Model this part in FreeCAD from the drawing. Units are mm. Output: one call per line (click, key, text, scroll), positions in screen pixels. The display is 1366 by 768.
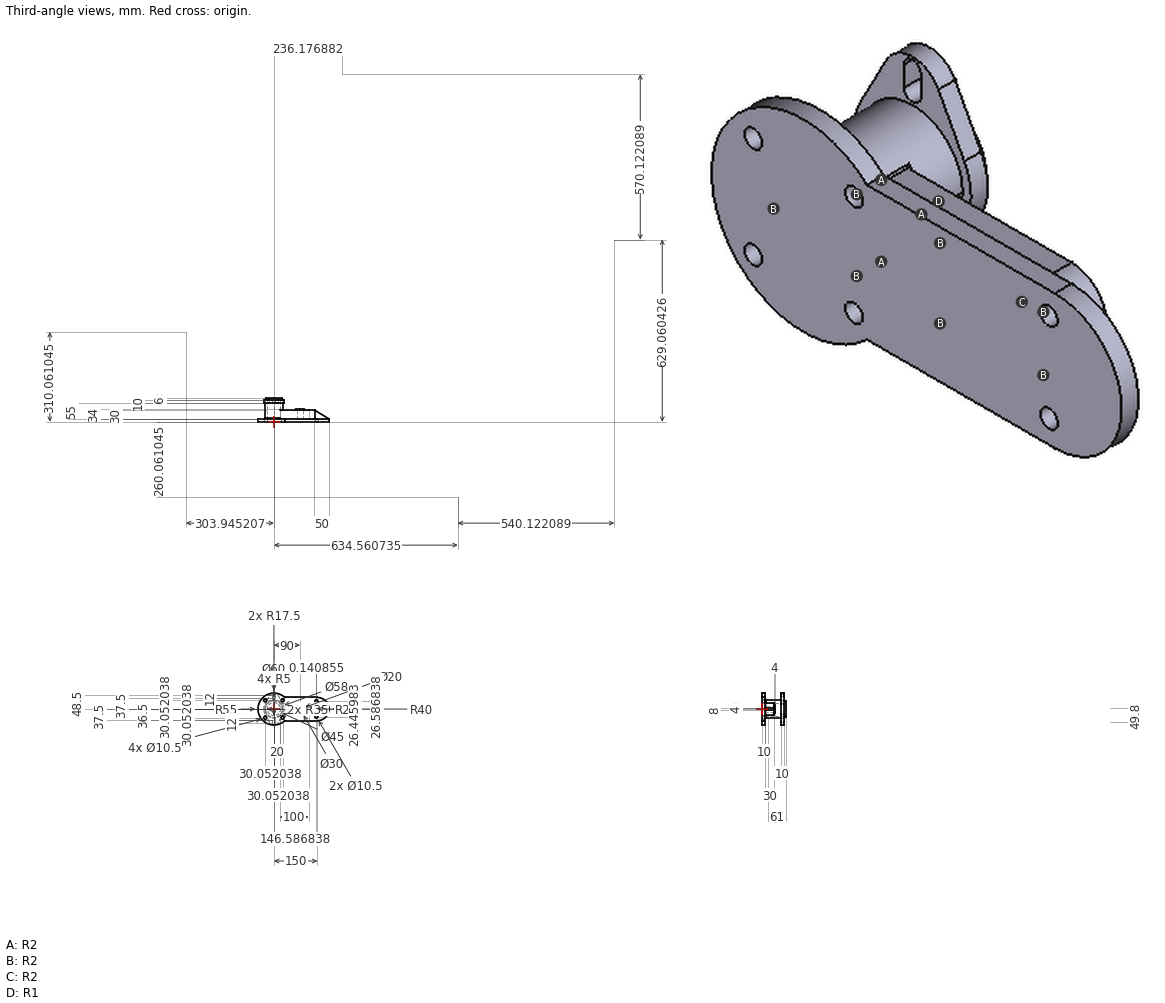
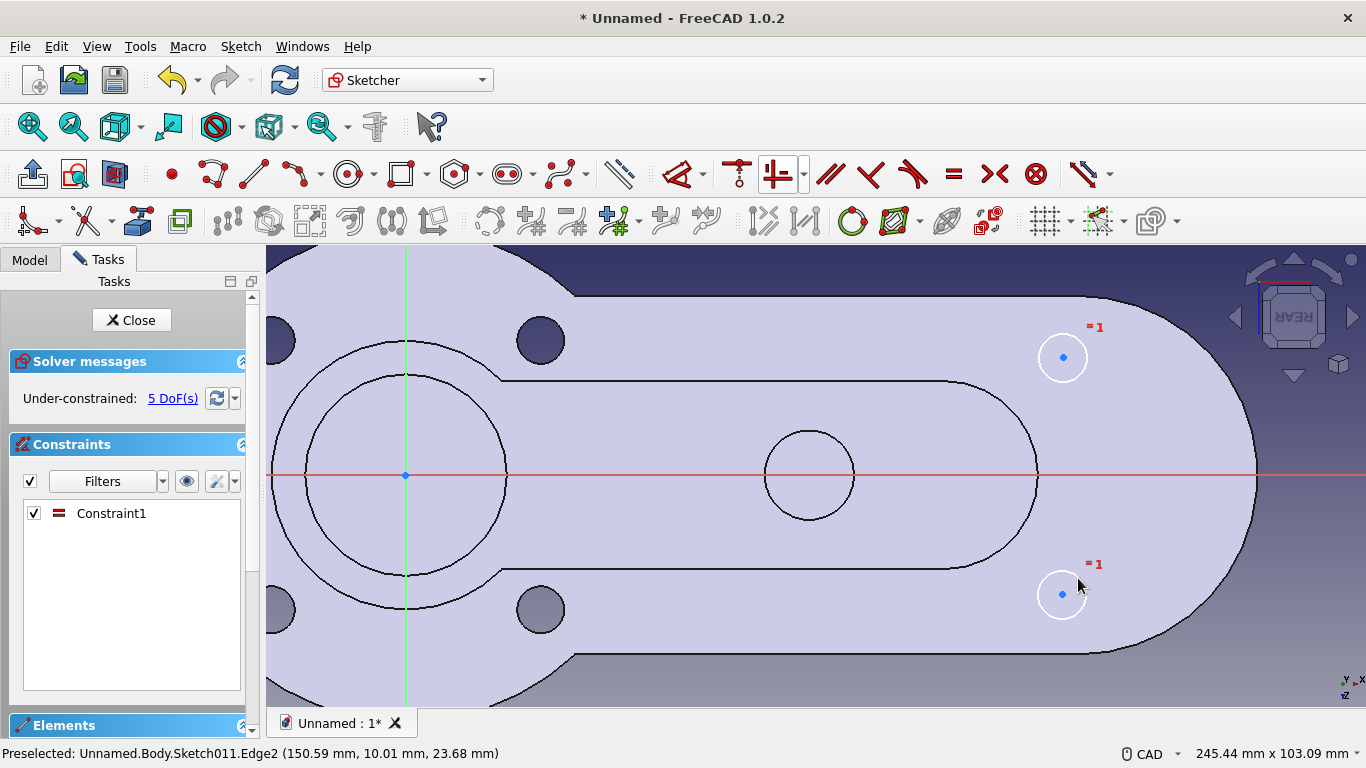
key(d)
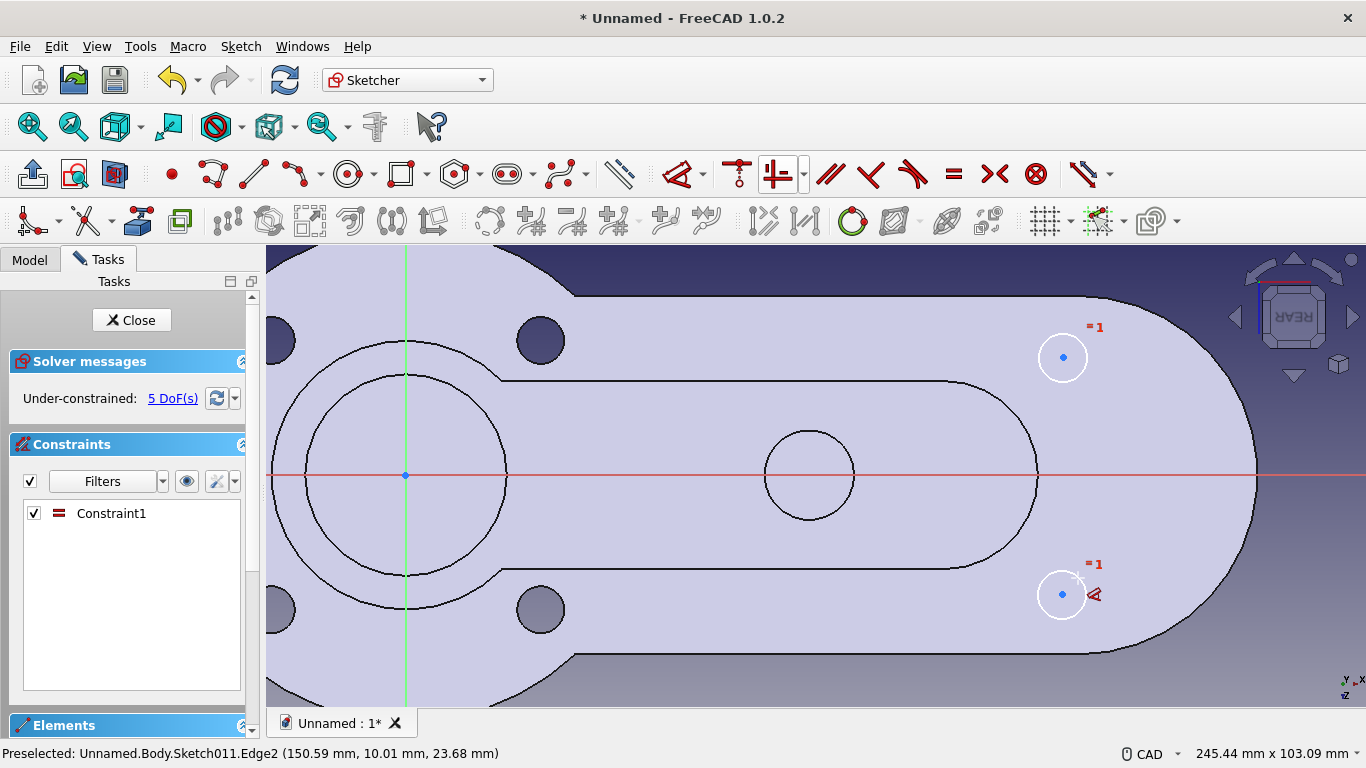
click(1080, 341)
click(1103, 318)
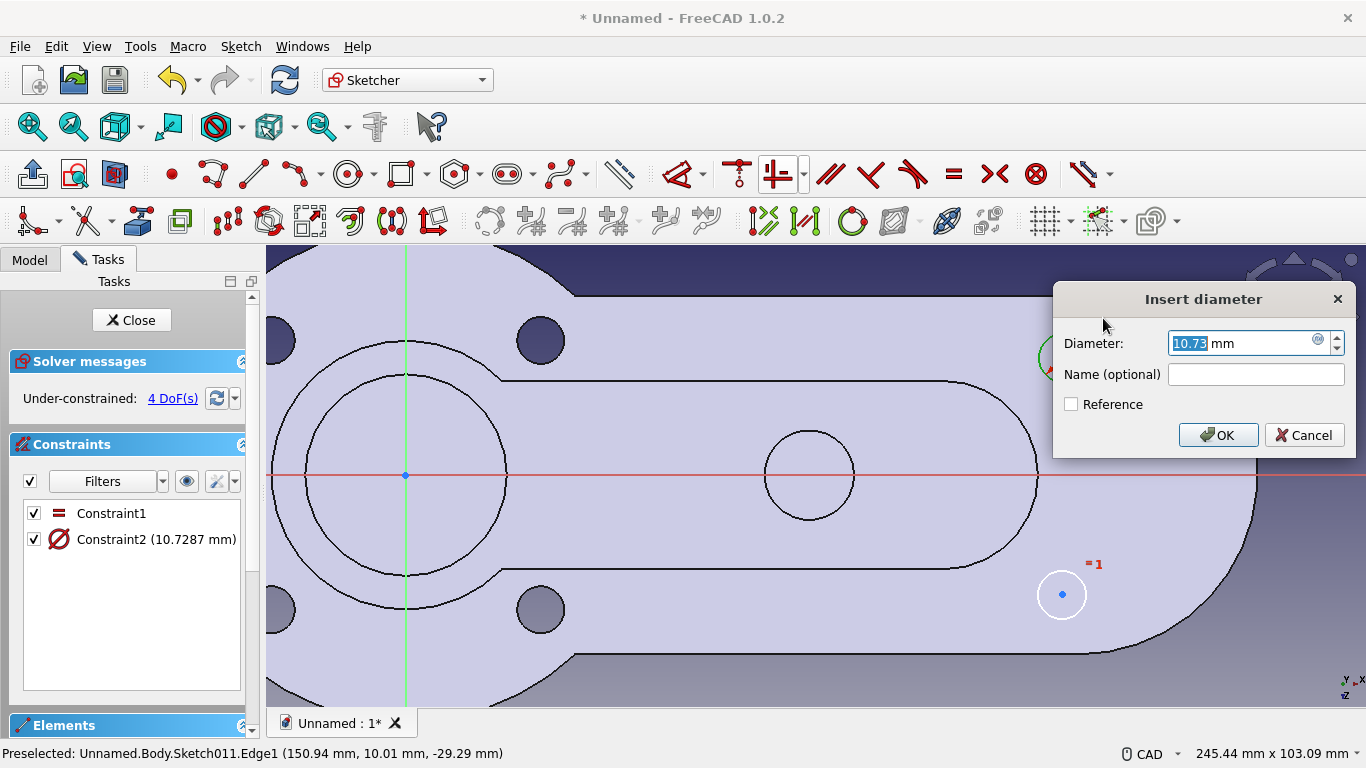
text(10.5)
key(Return)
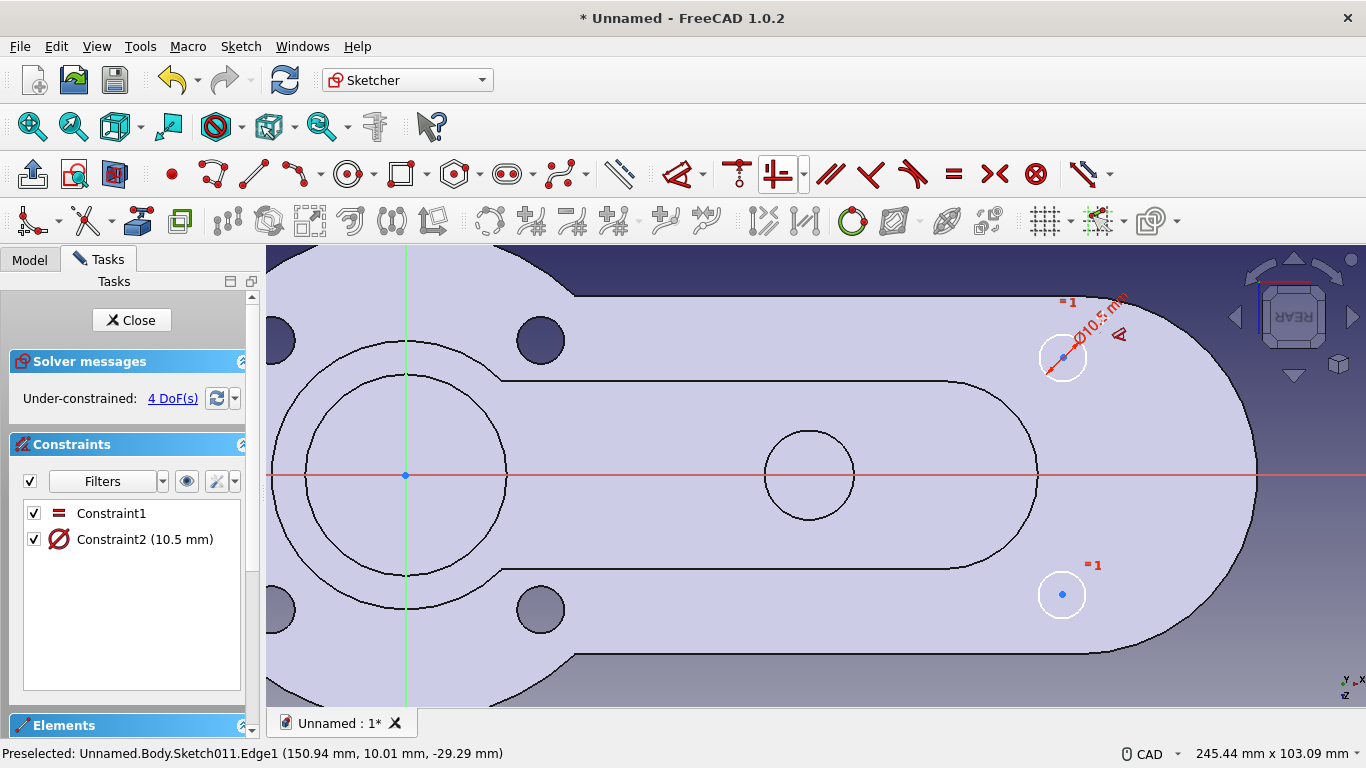
click(1063, 358)
click(372, 417)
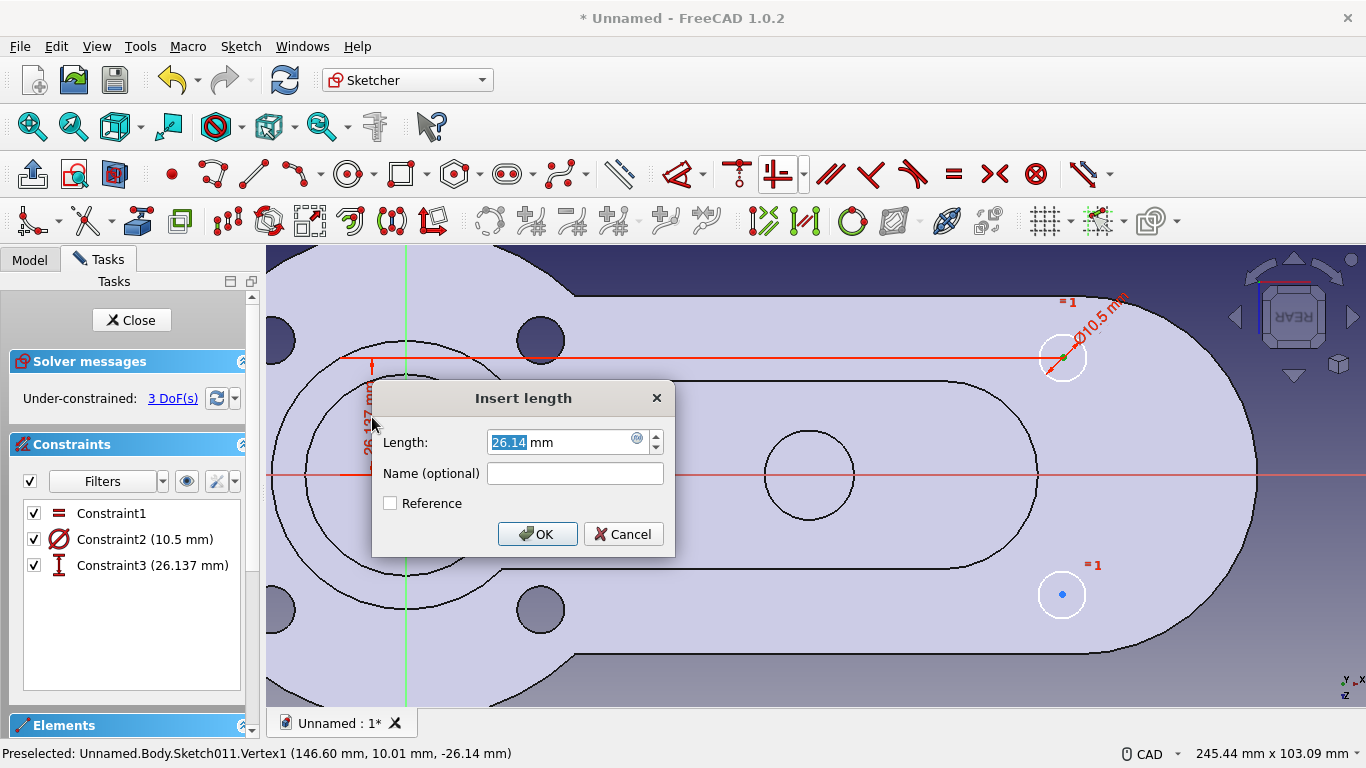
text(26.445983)
key(Return)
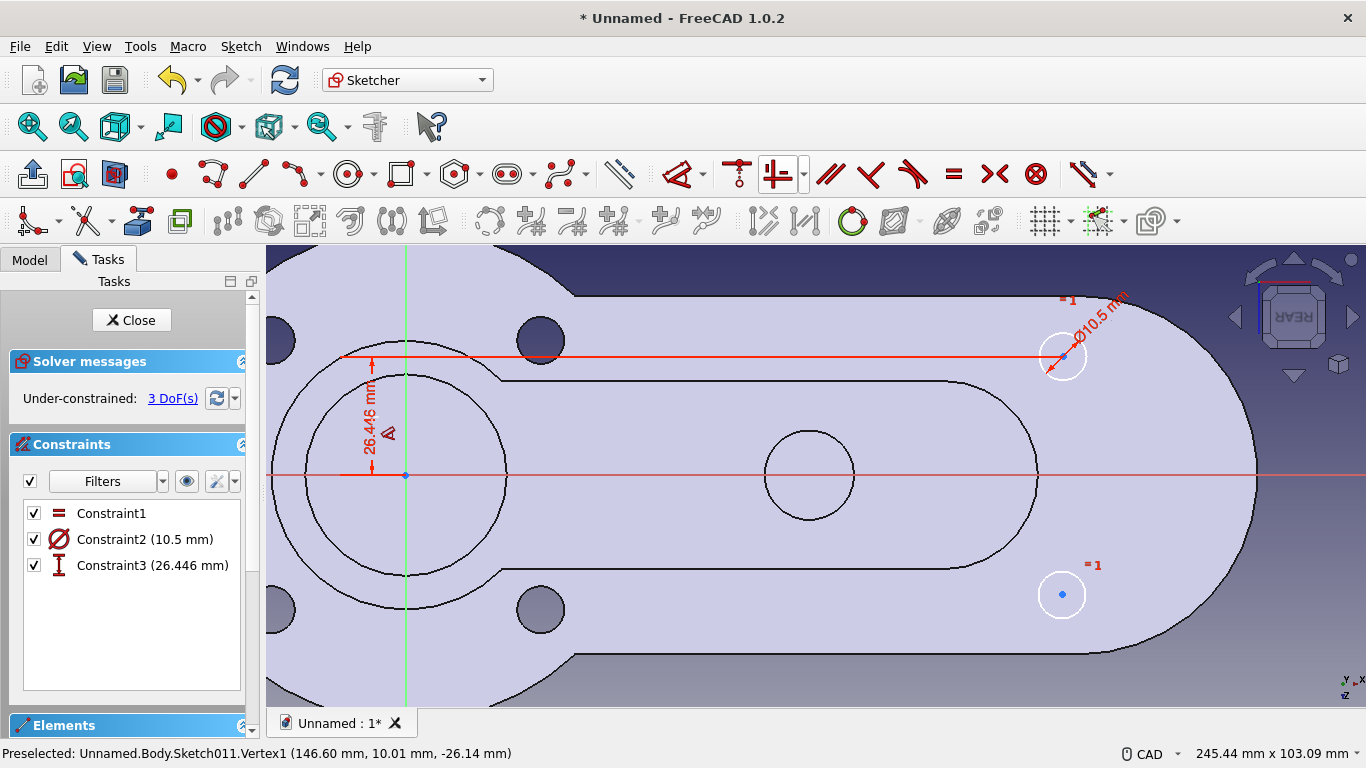
click(1062, 595)
click(372, 535)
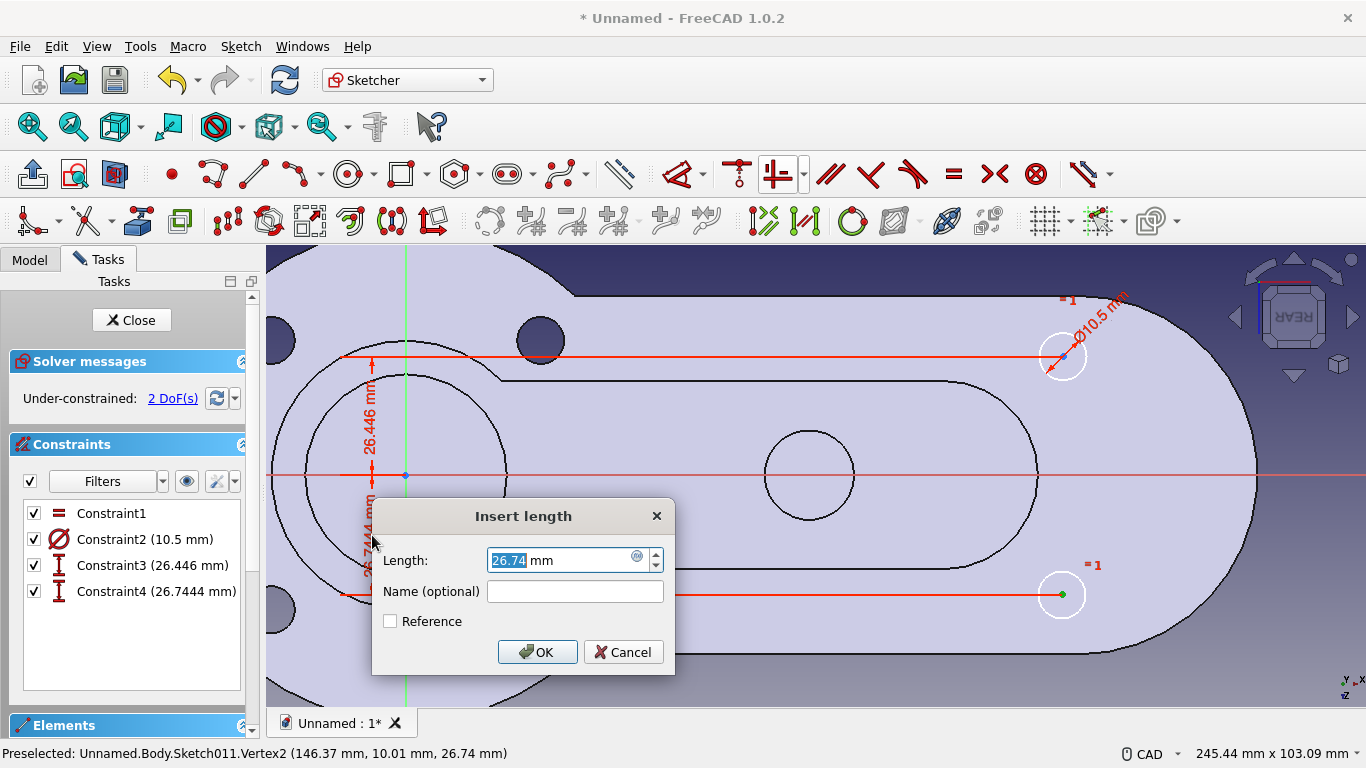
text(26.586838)
key(Return)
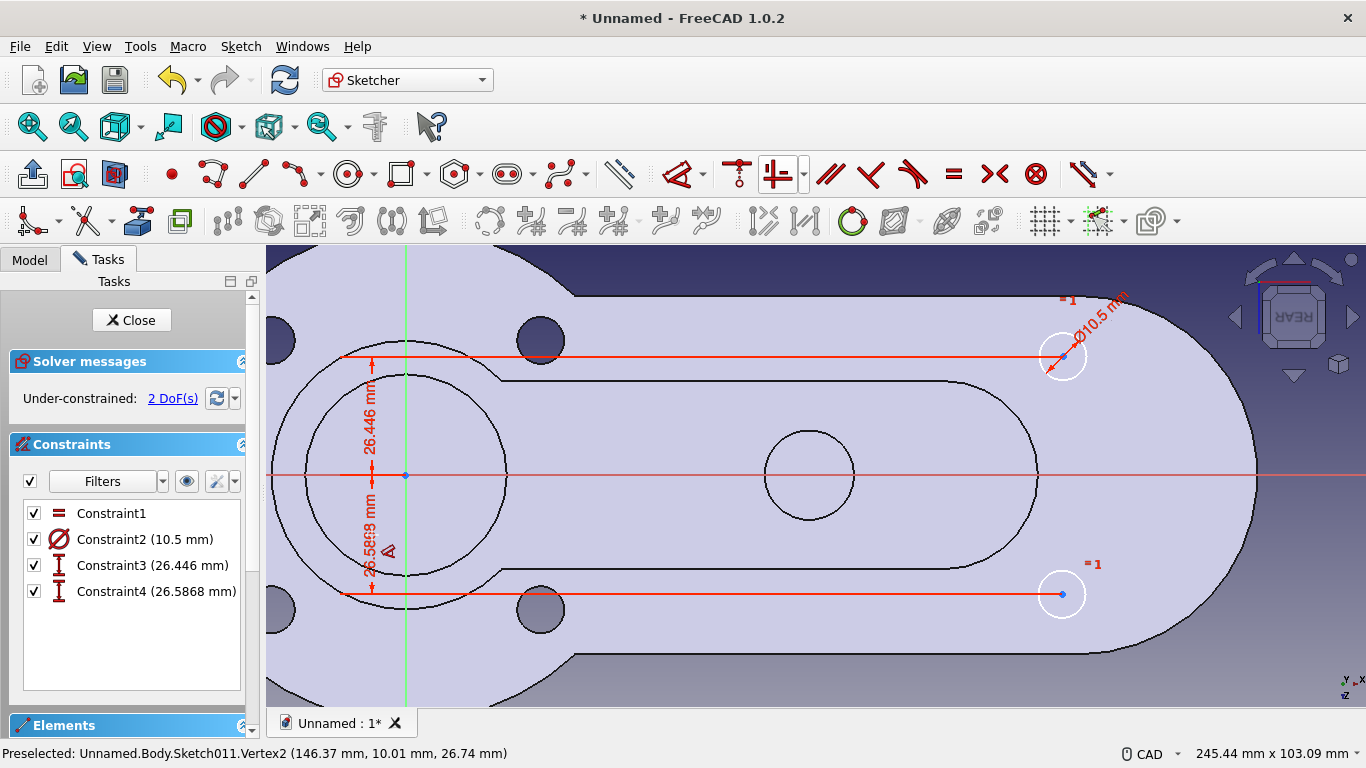
scroll(1063, 357, up, 21)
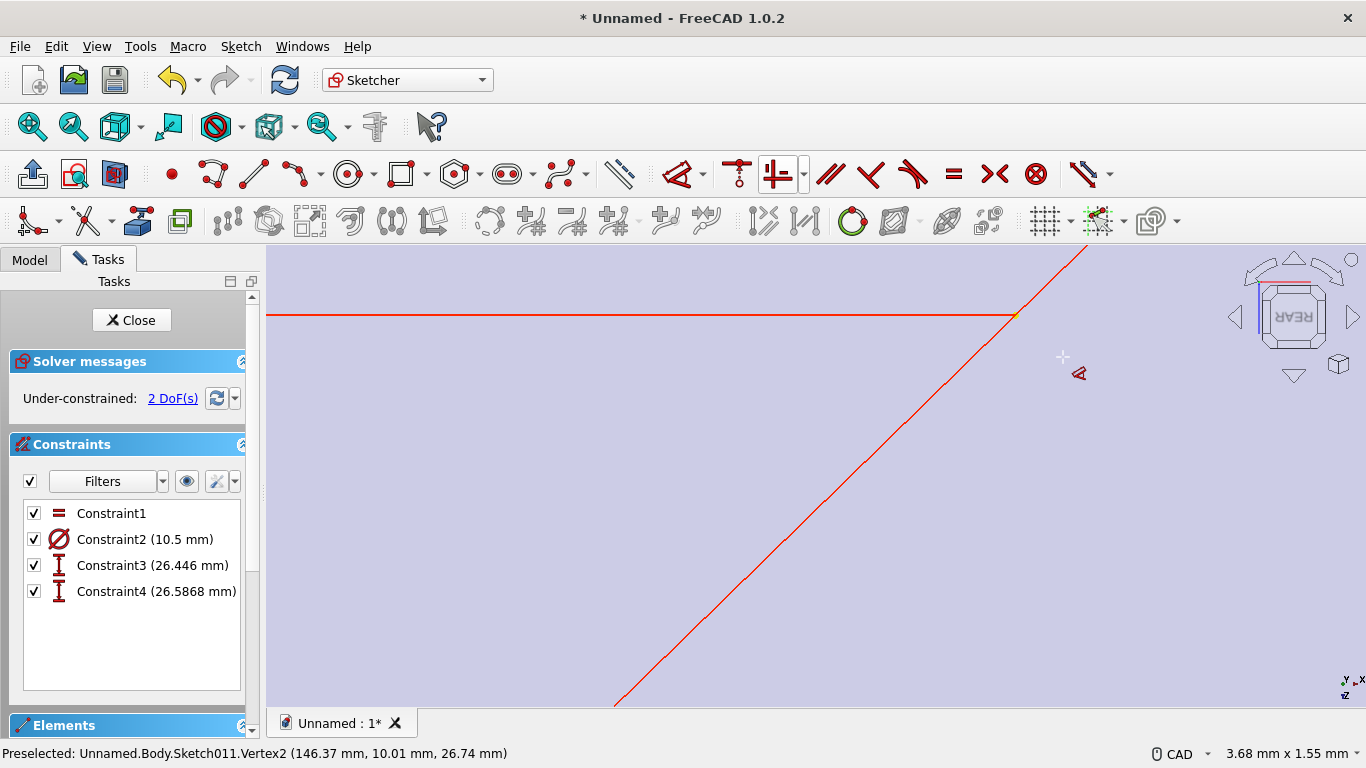
click(1015, 315)